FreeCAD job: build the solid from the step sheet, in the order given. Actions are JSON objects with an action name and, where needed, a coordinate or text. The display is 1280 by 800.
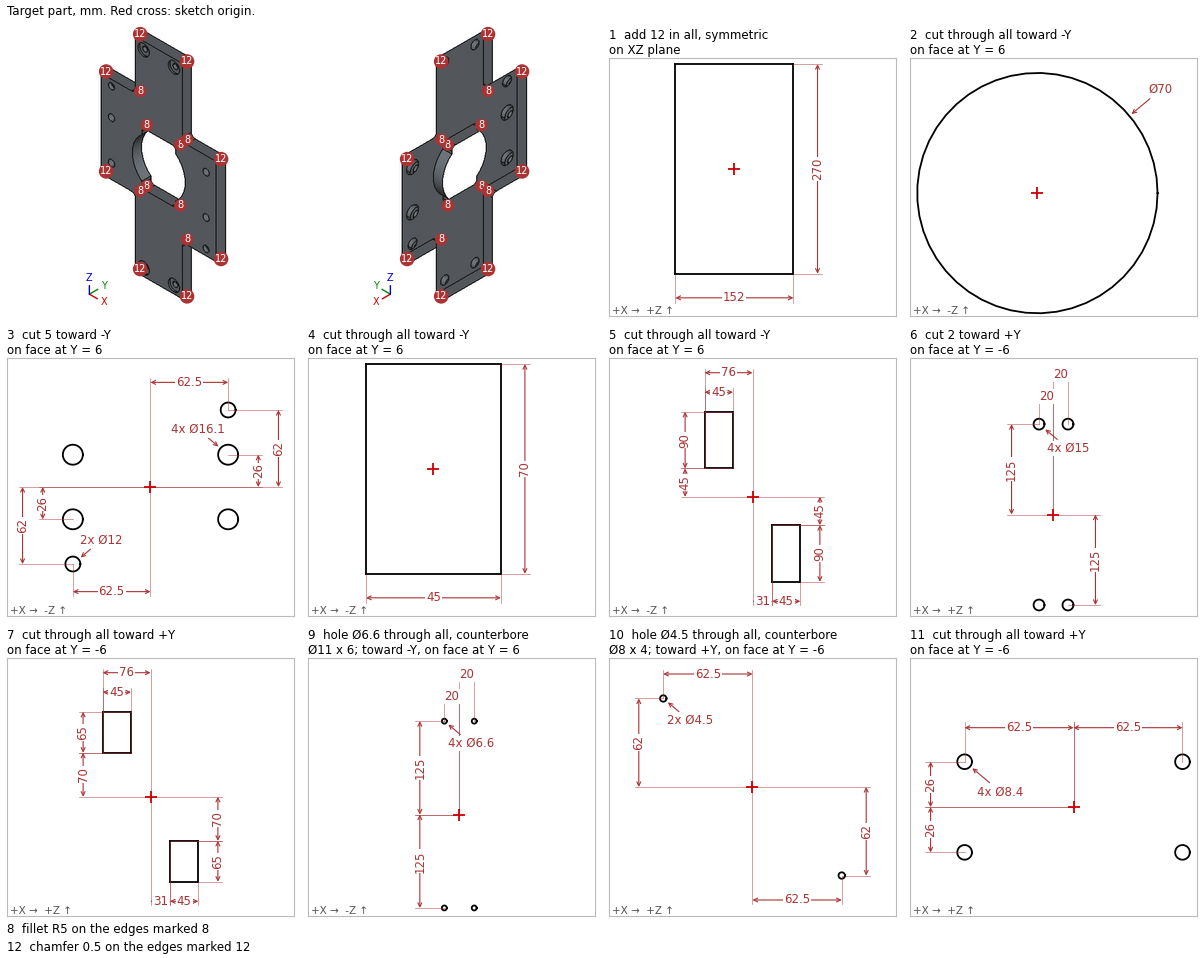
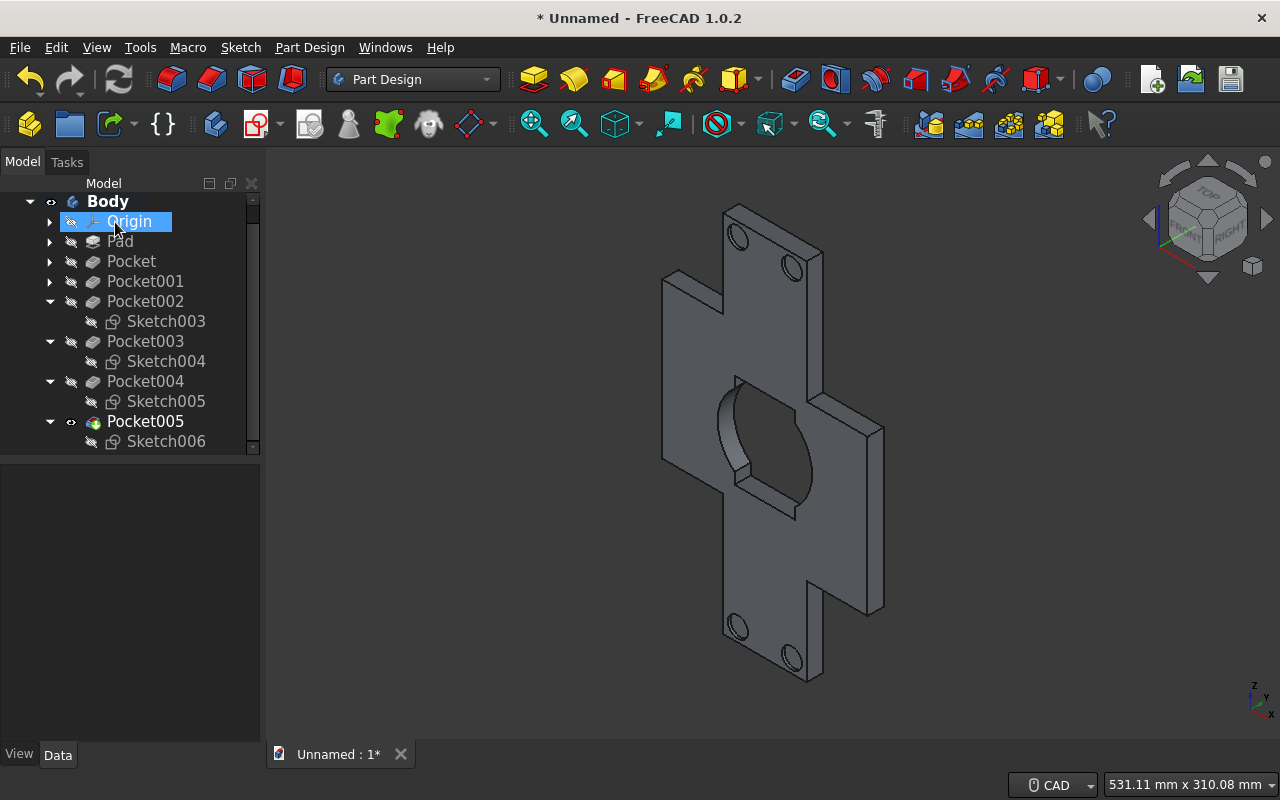
{"action": "key", "text": "1"}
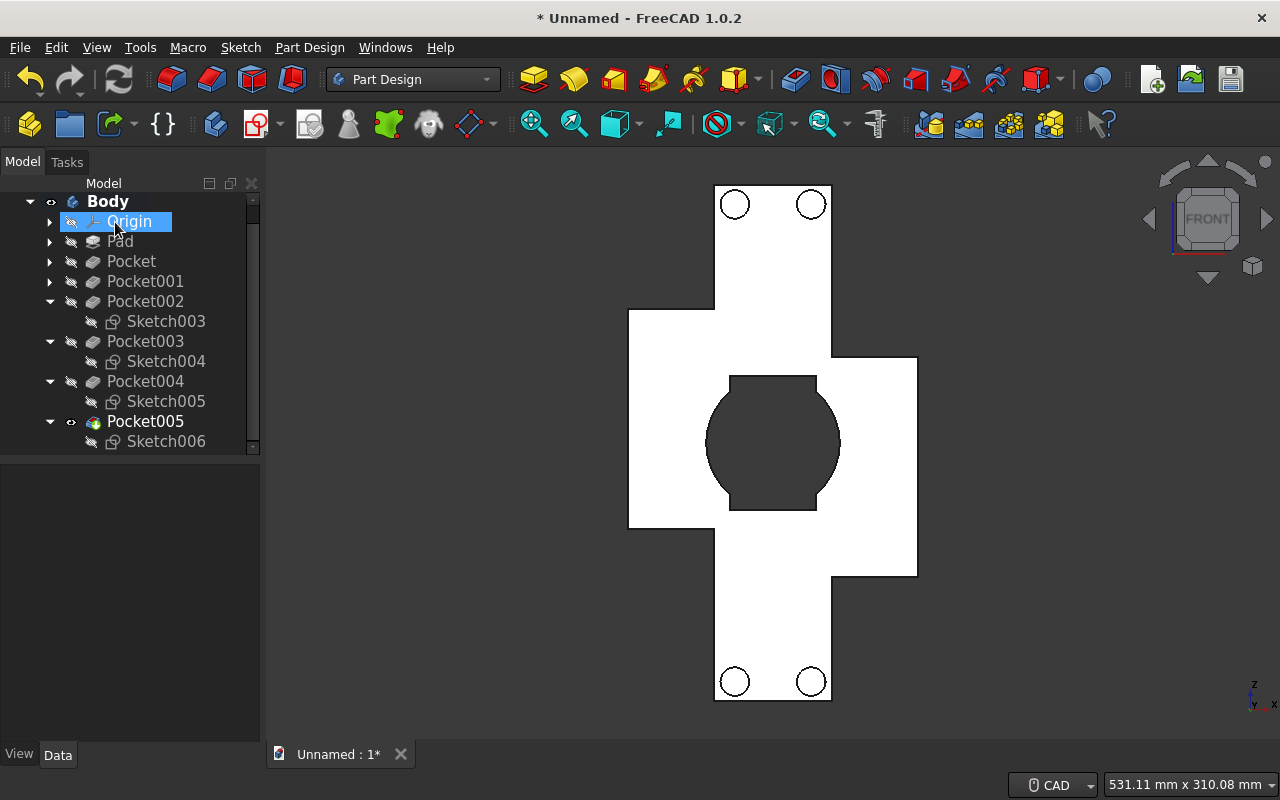
{"action": "key", "text": "3"}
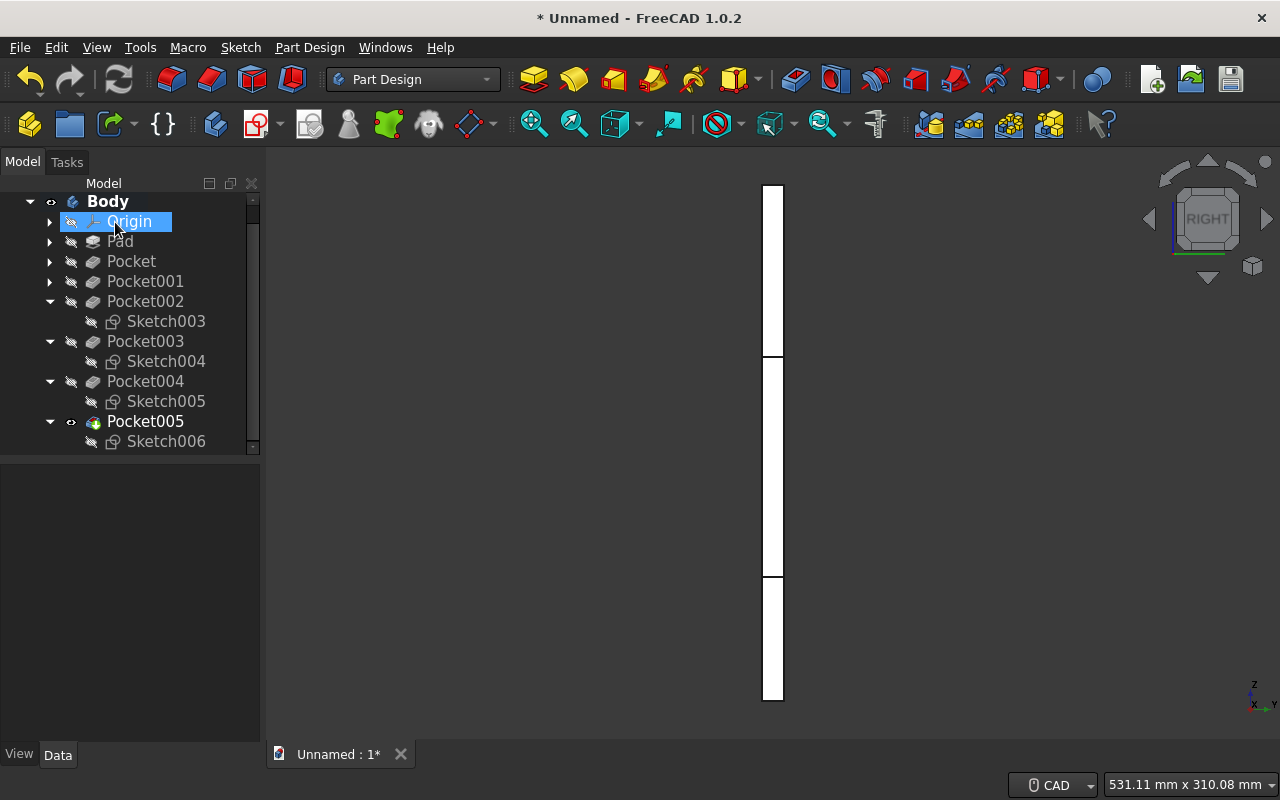
{"action": "key", "text": "5"}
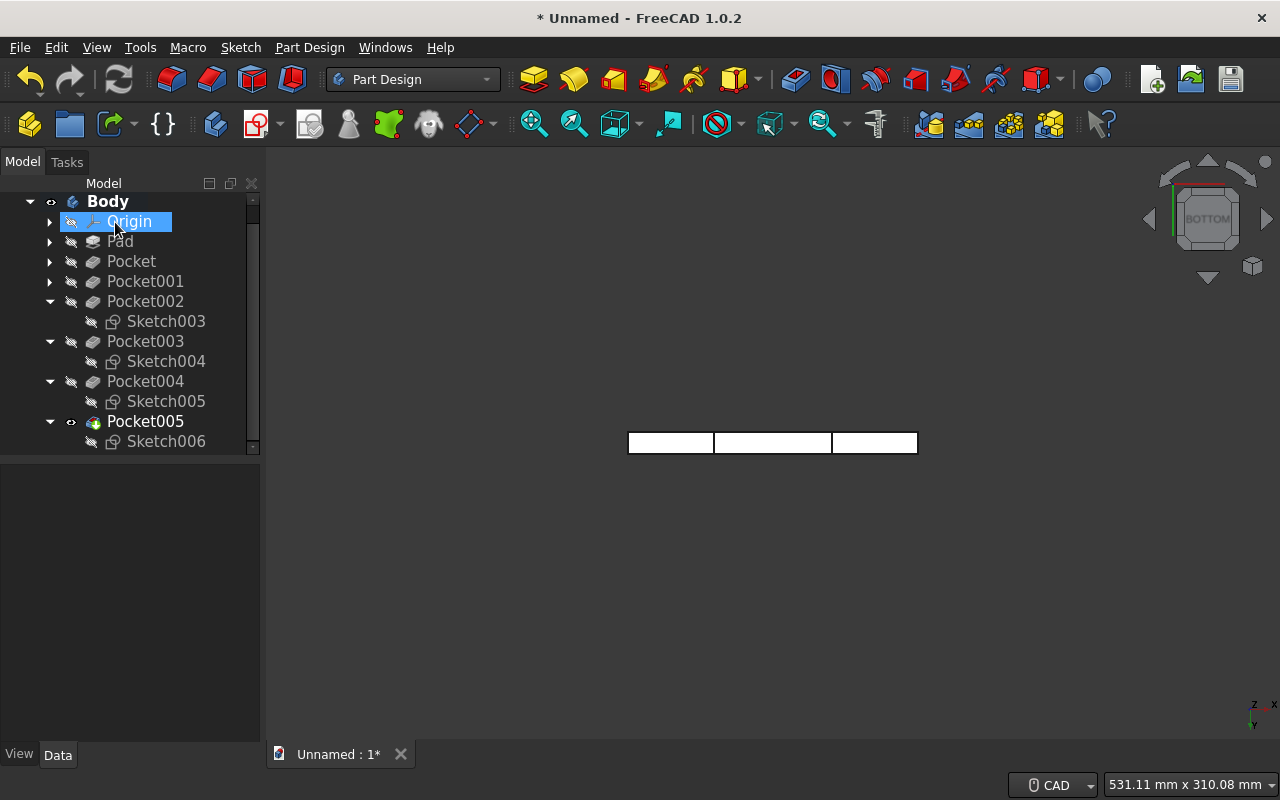
{"action": "key", "text": "v f"}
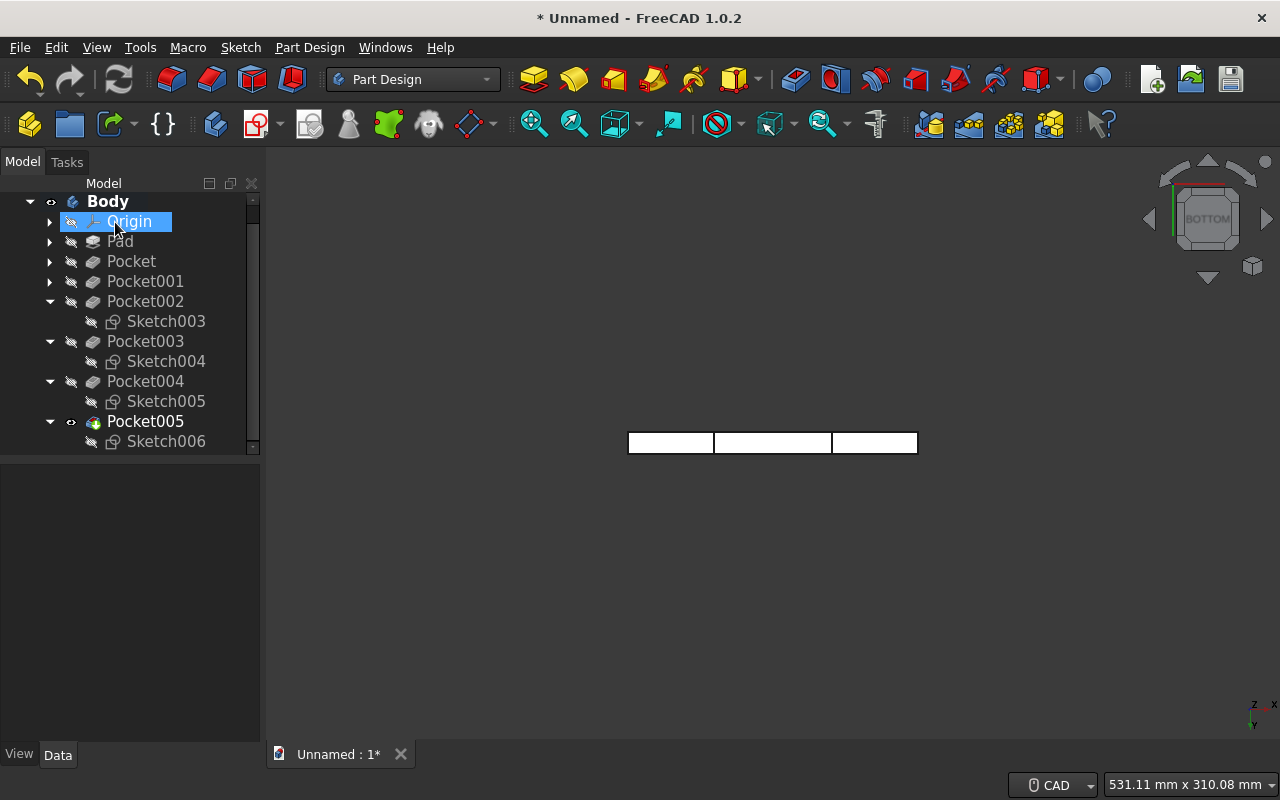
{"action": "key", "text": "4"}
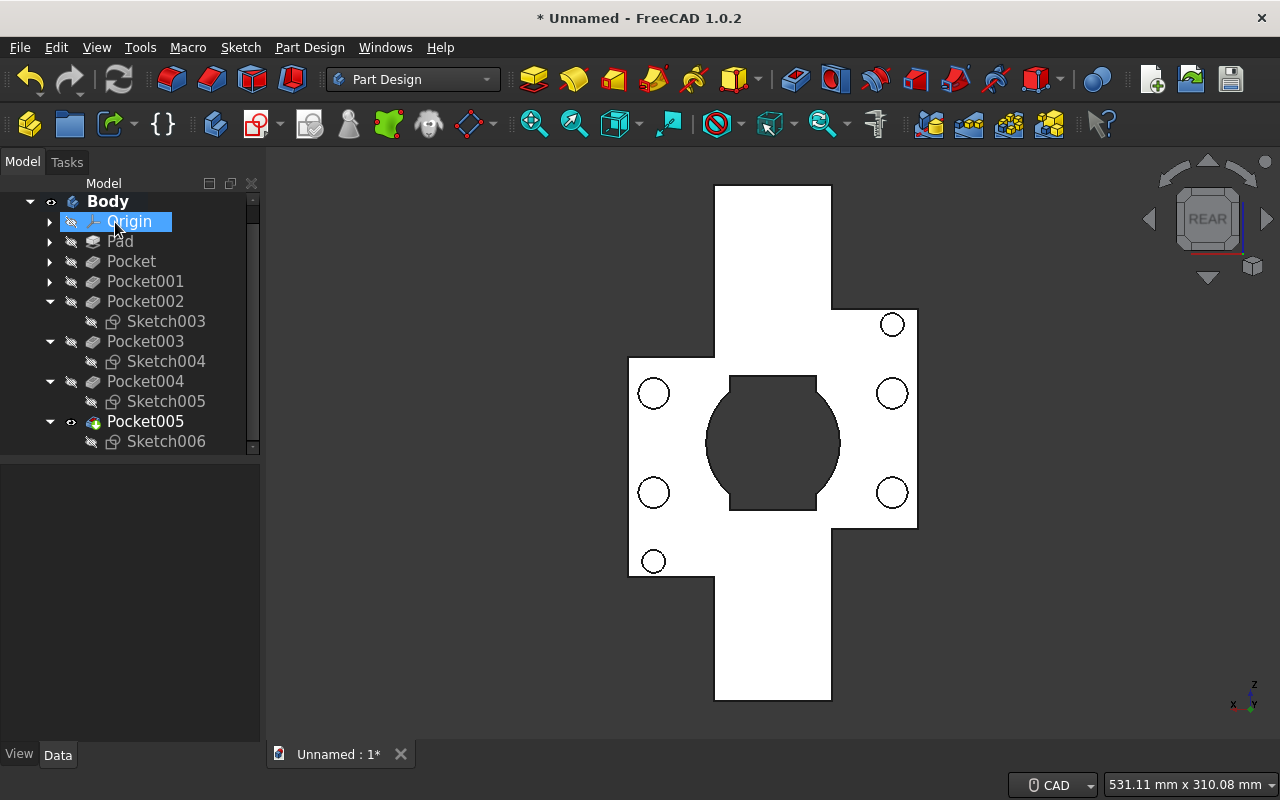
{"action": "key", "text": "6"}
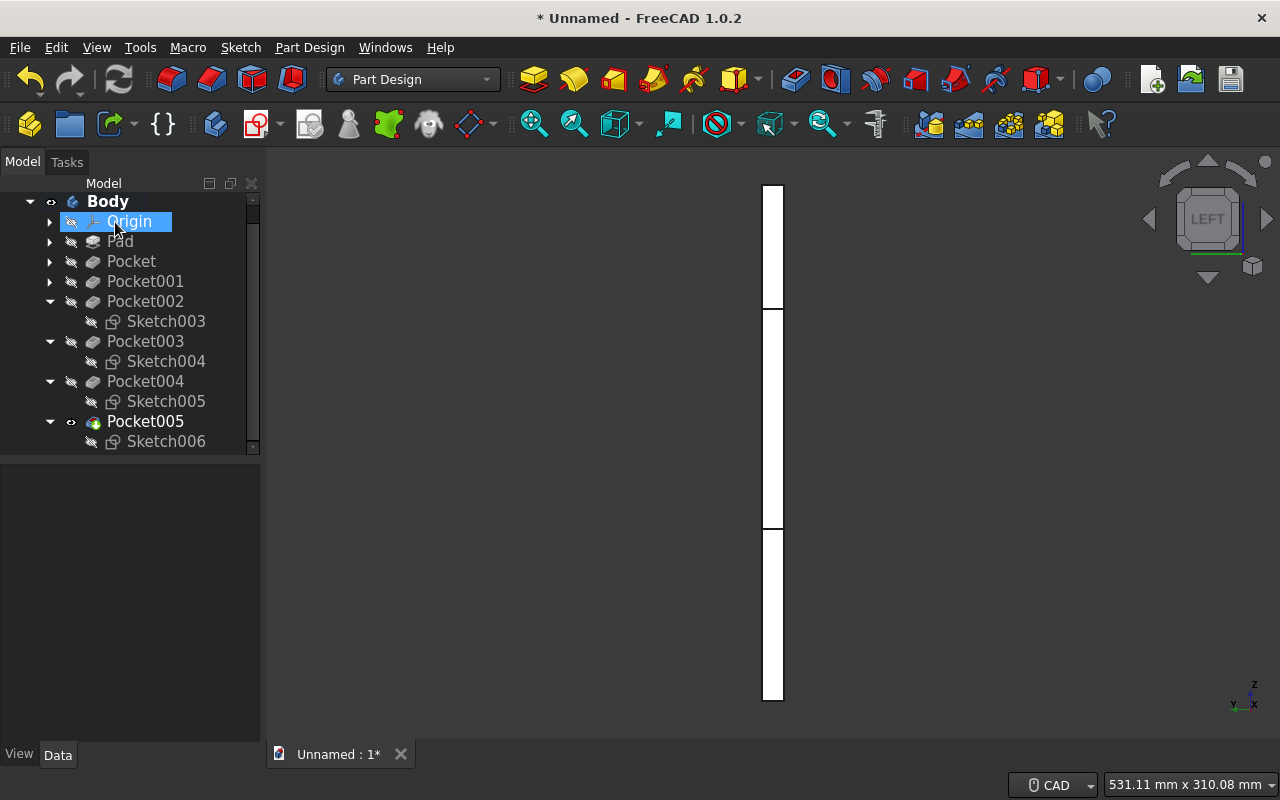
{"action": "key", "text": "v 3"}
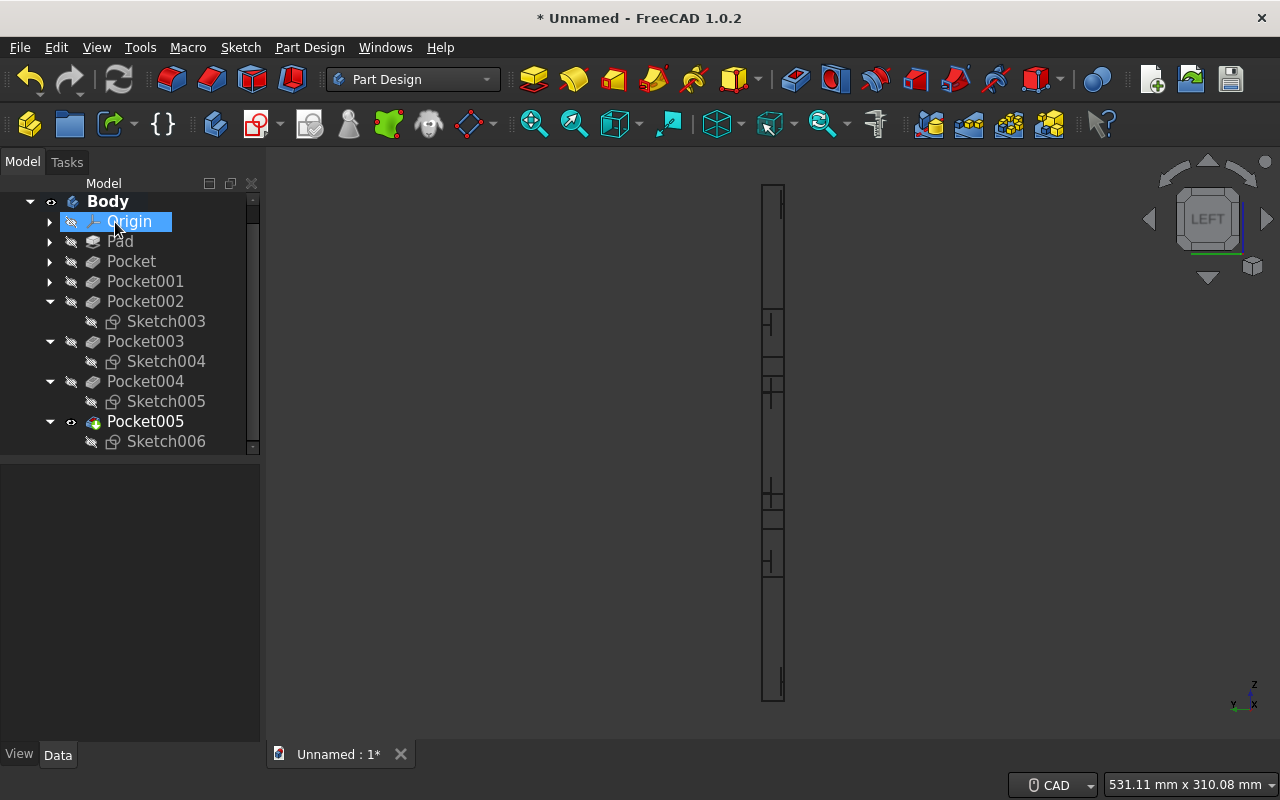
{"action": "key", "text": "0"}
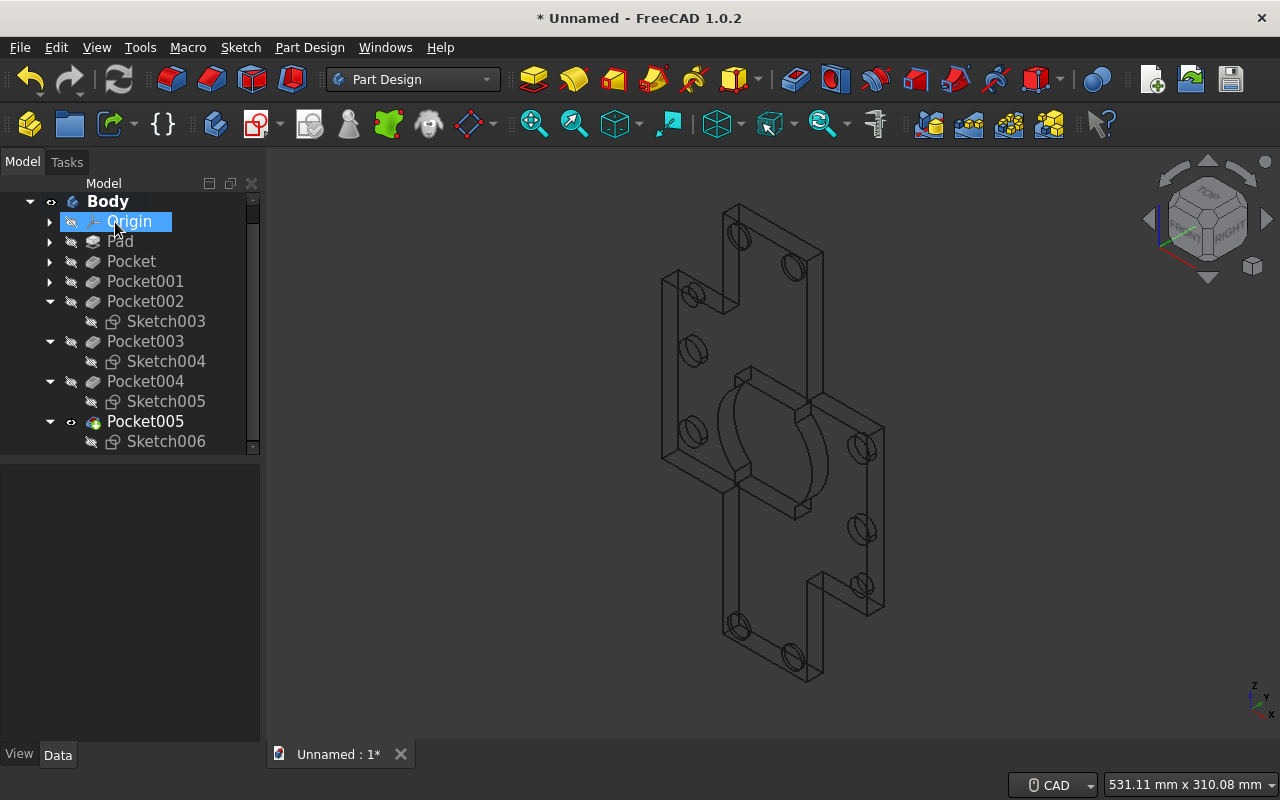
{"action": "left_click", "coordinate": [731, 309]}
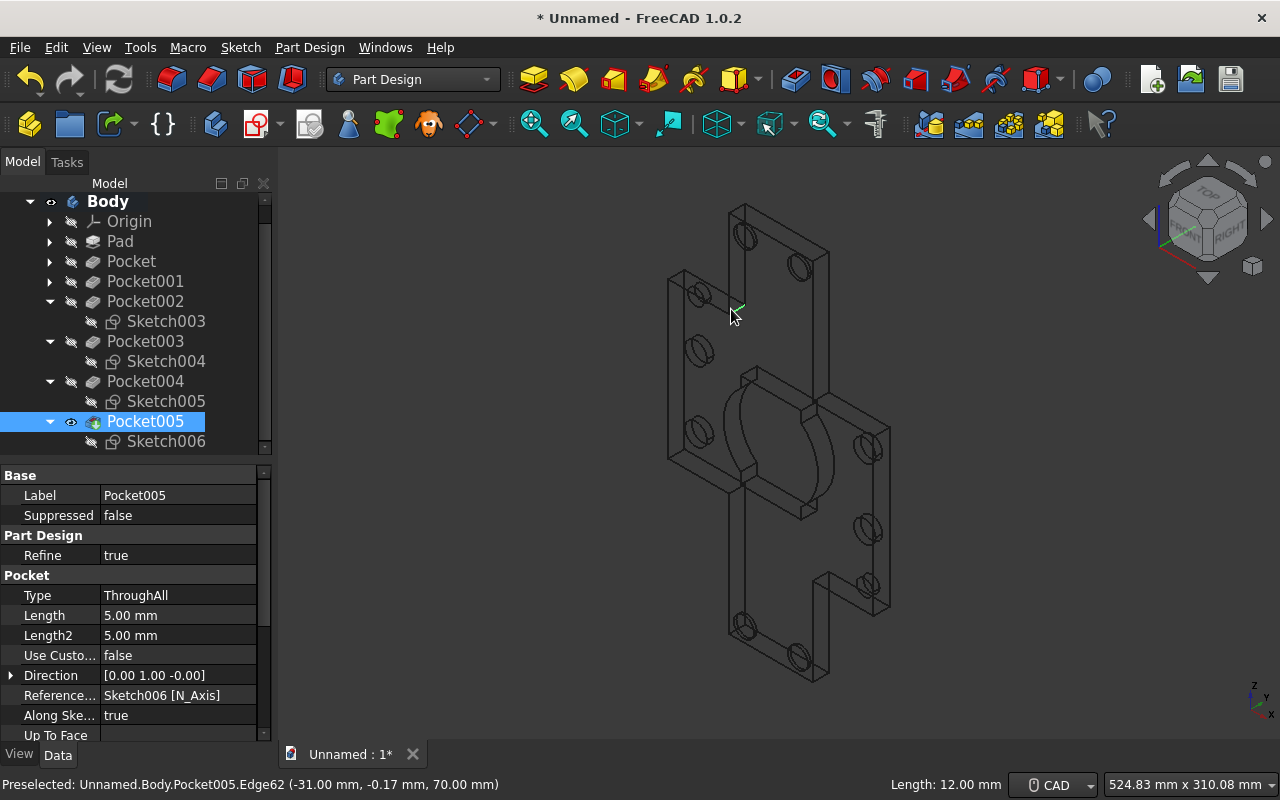
{"action": "left_click", "coordinate": [821, 575], "text": "ctrl"}